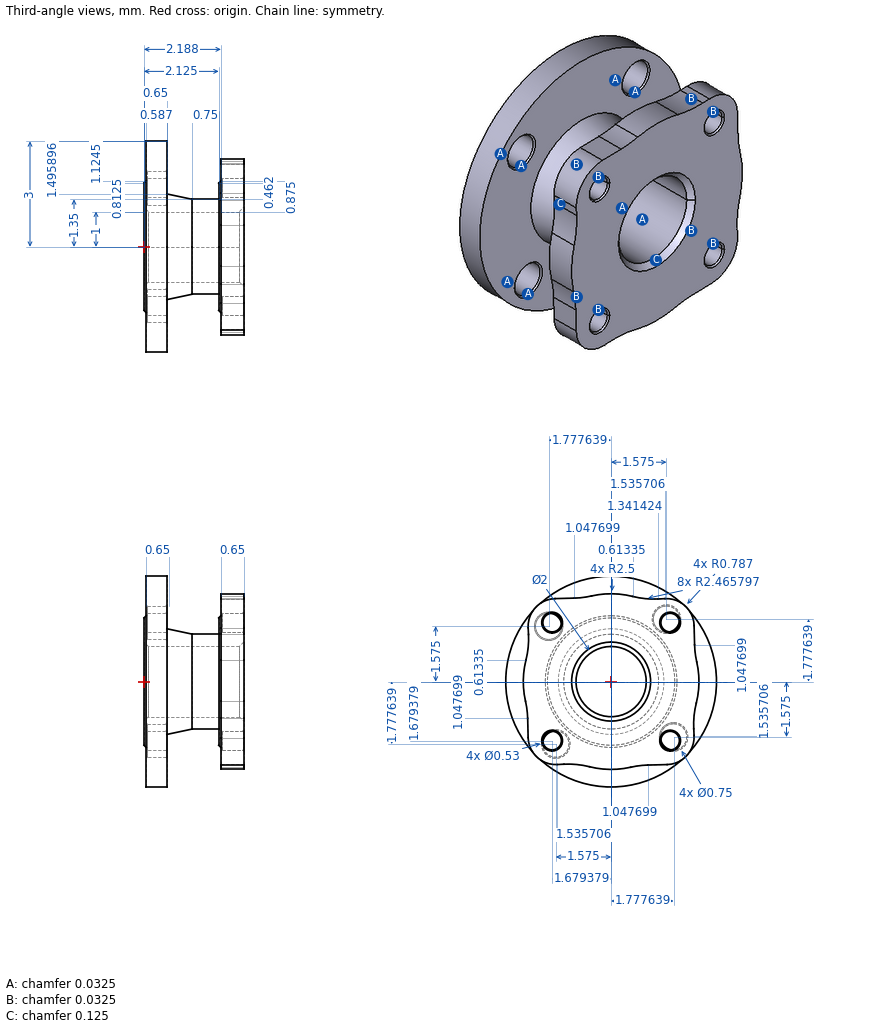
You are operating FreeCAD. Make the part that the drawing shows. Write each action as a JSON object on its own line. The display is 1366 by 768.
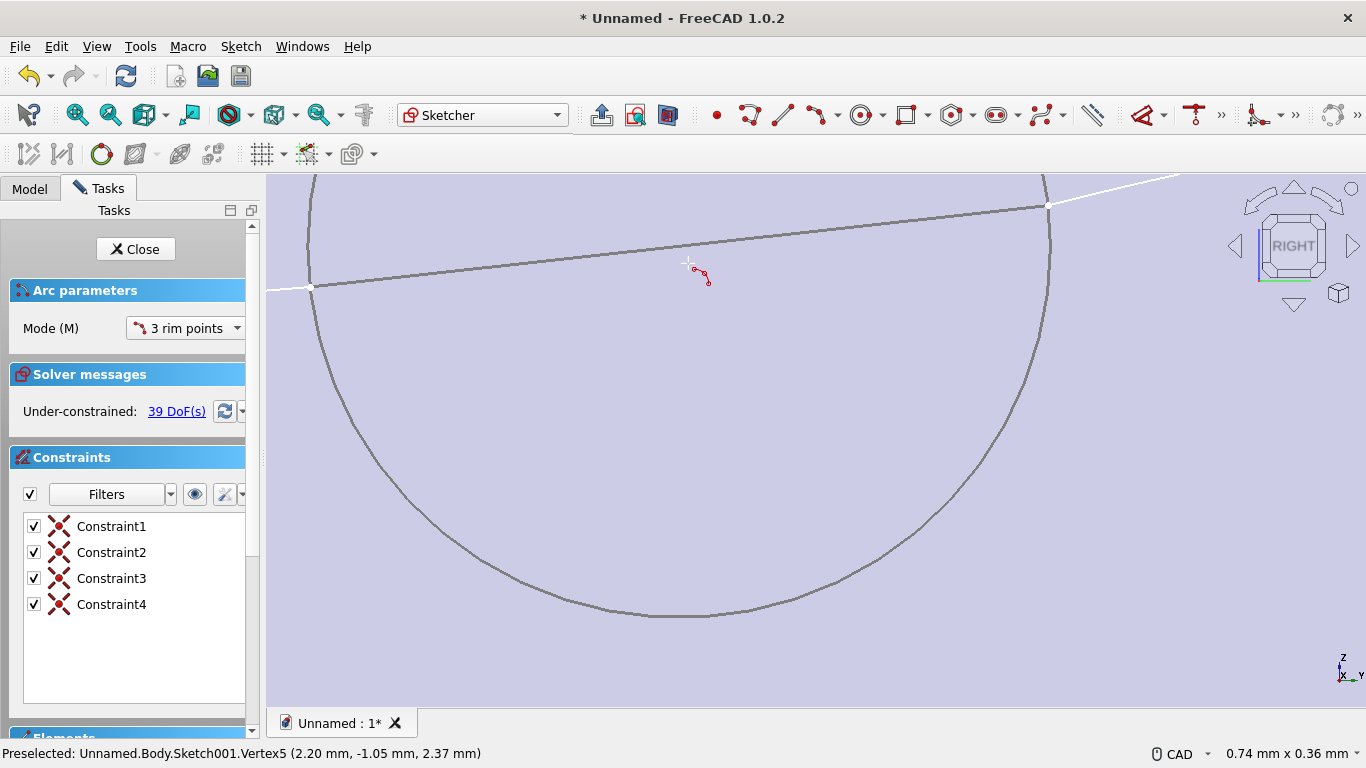
{"action": "left_click", "coordinate": [683, 250]}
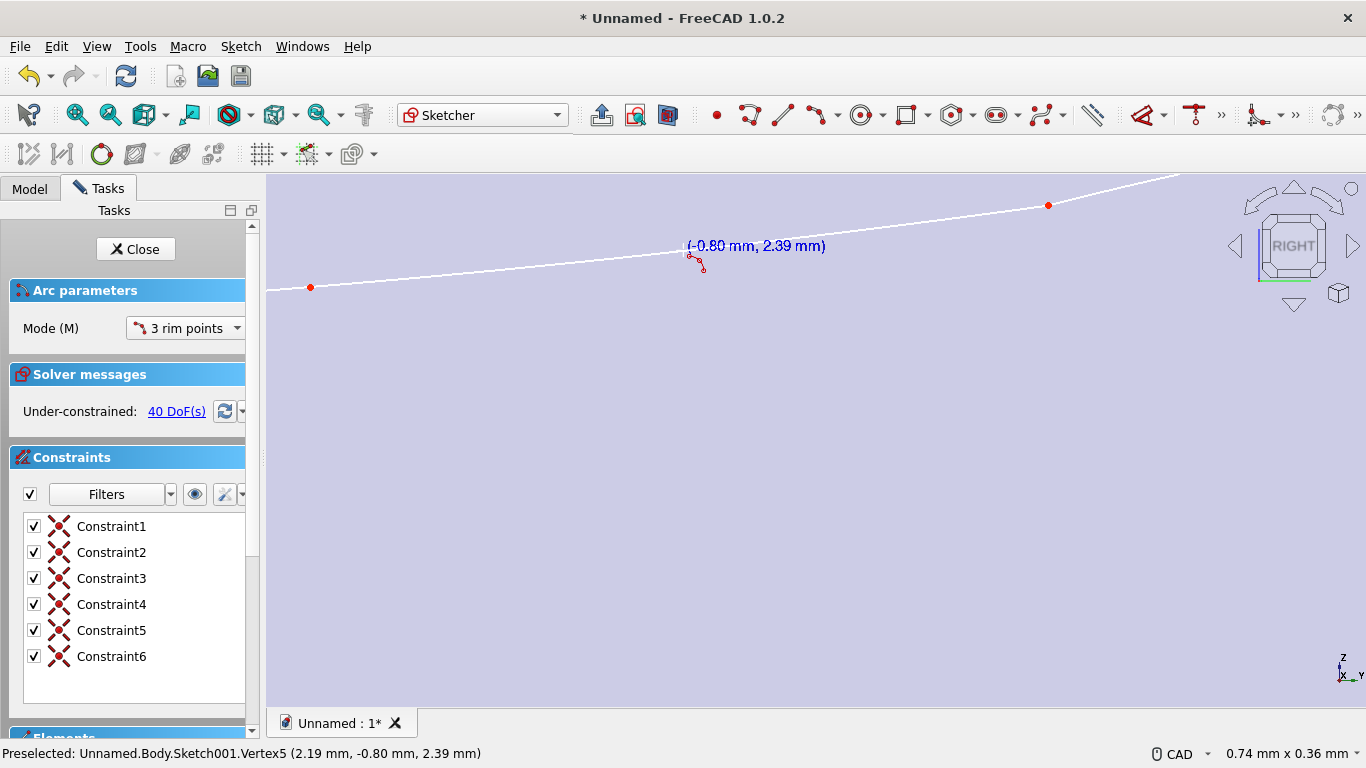
{"action": "scroll", "coordinate": [688, 263], "scroll_direction": "down", "scroll_amount": 15}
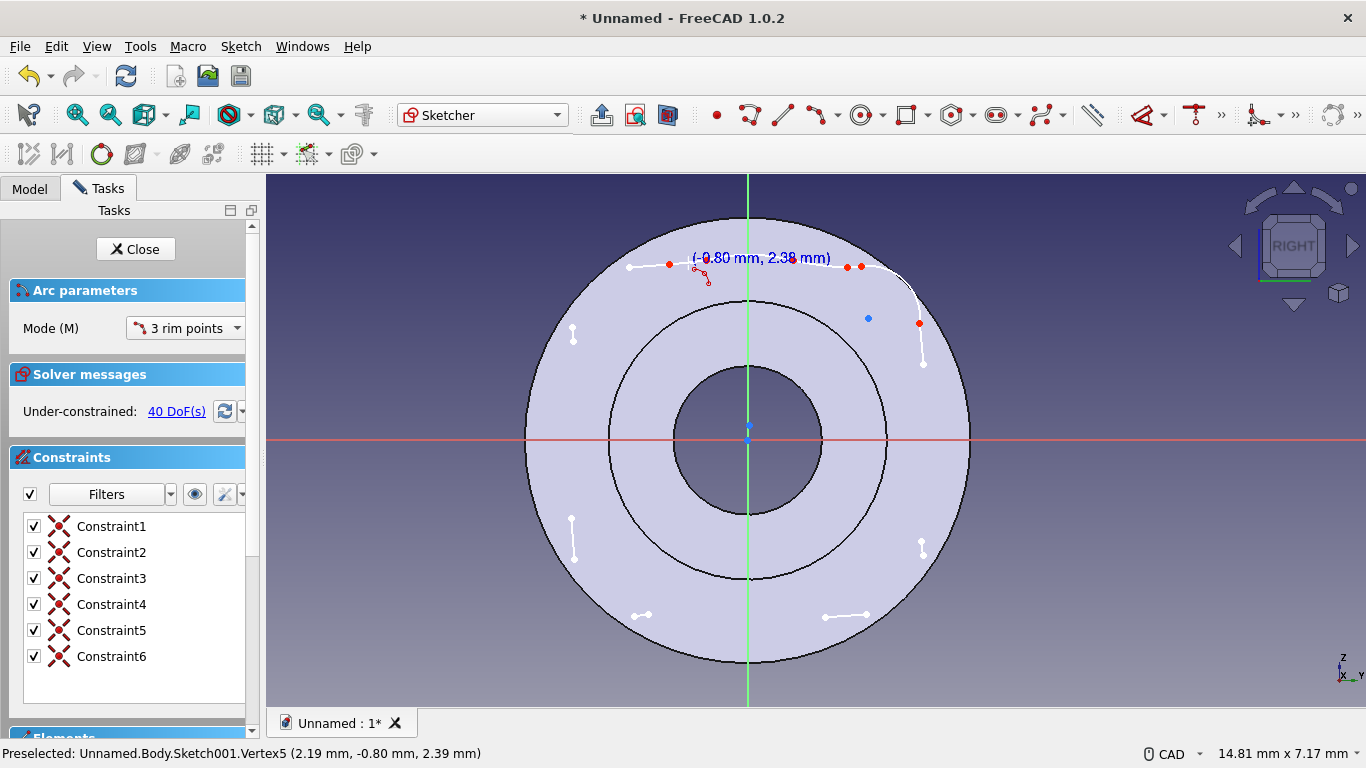
{"action": "left_click", "coordinate": [629, 268]}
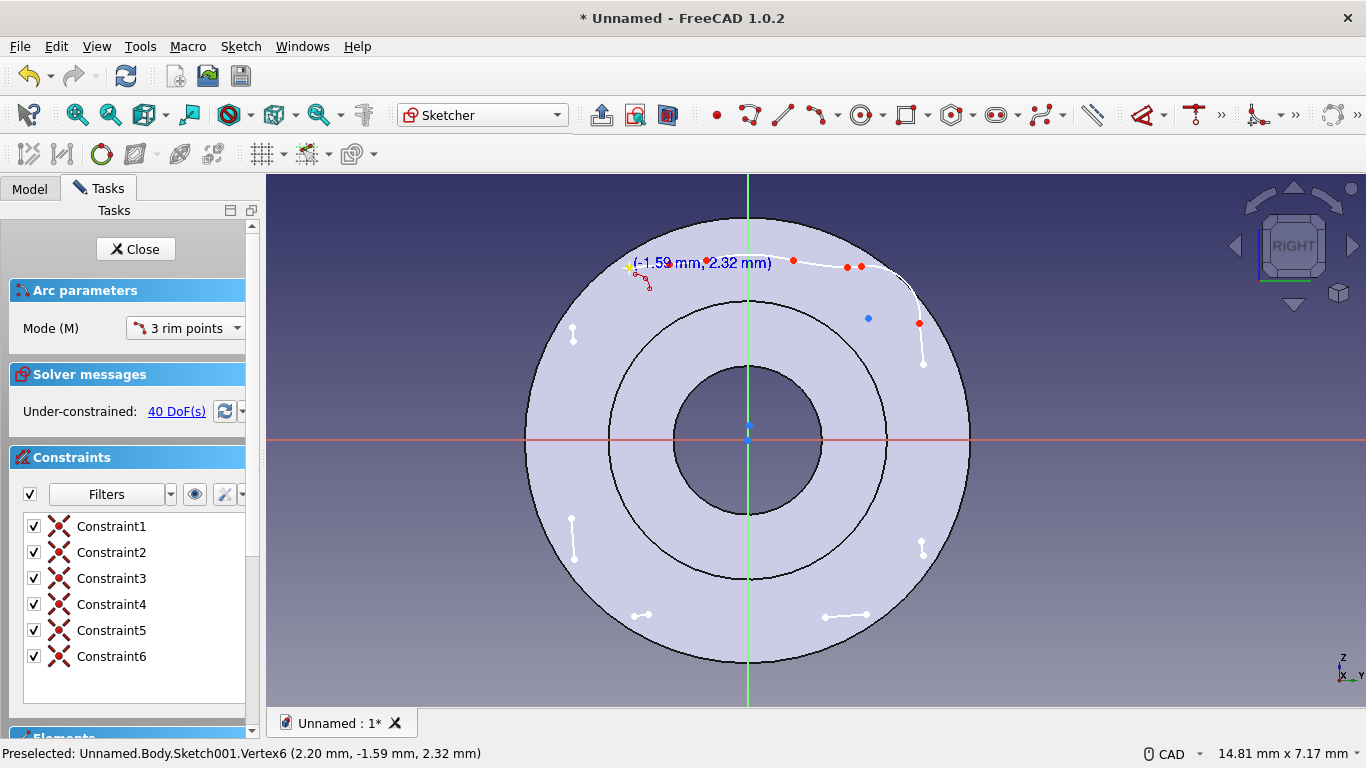
{"action": "scroll", "coordinate": [572, 326], "scroll_direction": "up", "scroll_amount": 4}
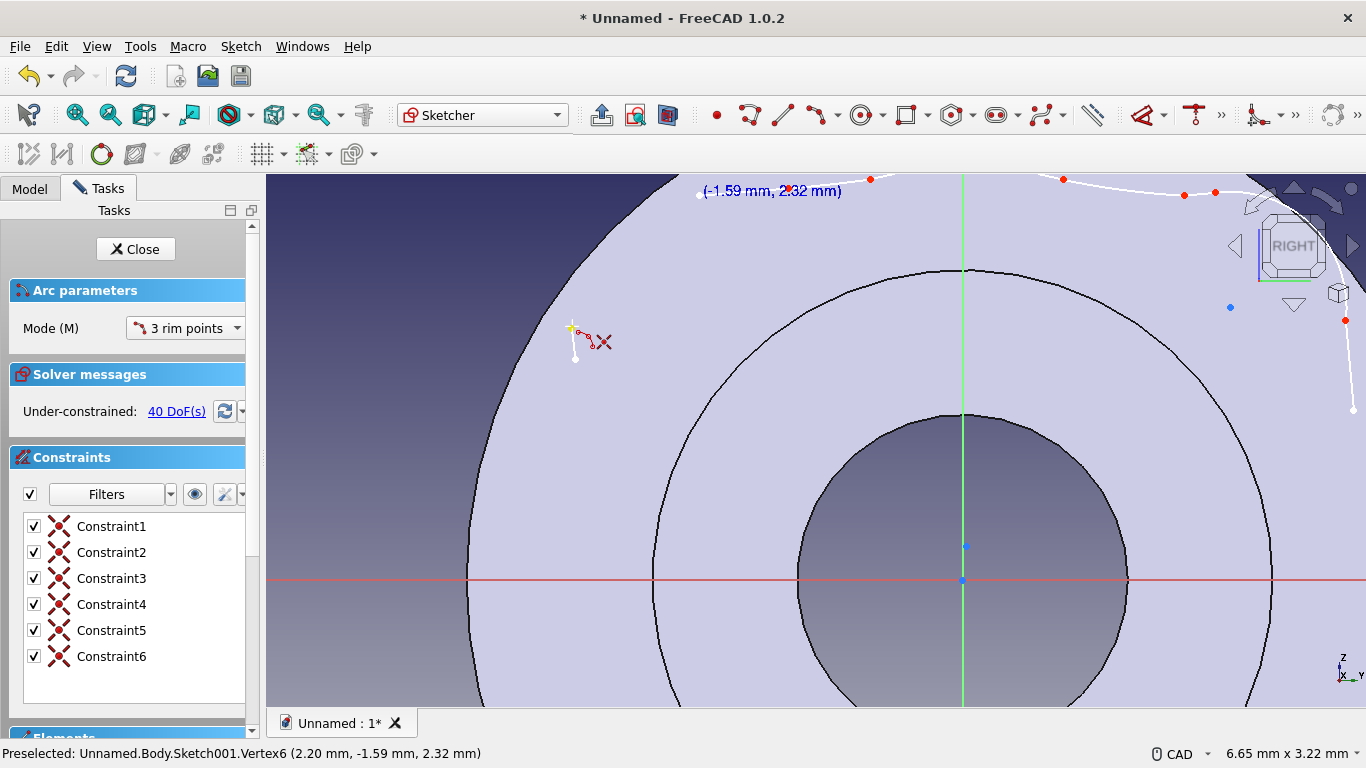
{"action": "left_click", "coordinate": [572, 329]}
{"action": "left_click", "coordinate": [607, 231]}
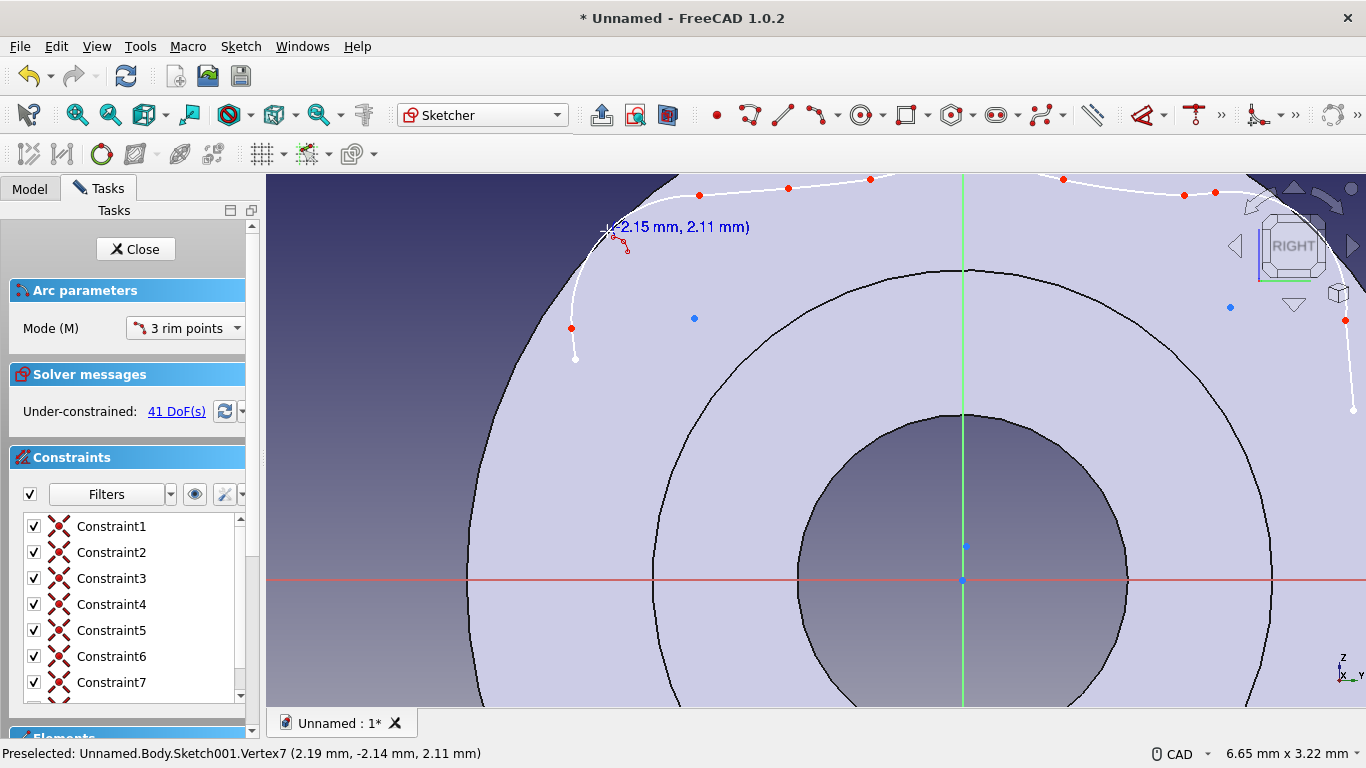
{"action": "left_click", "coordinate": [576, 360]}
{"action": "left_click", "coordinate": [562, 479]}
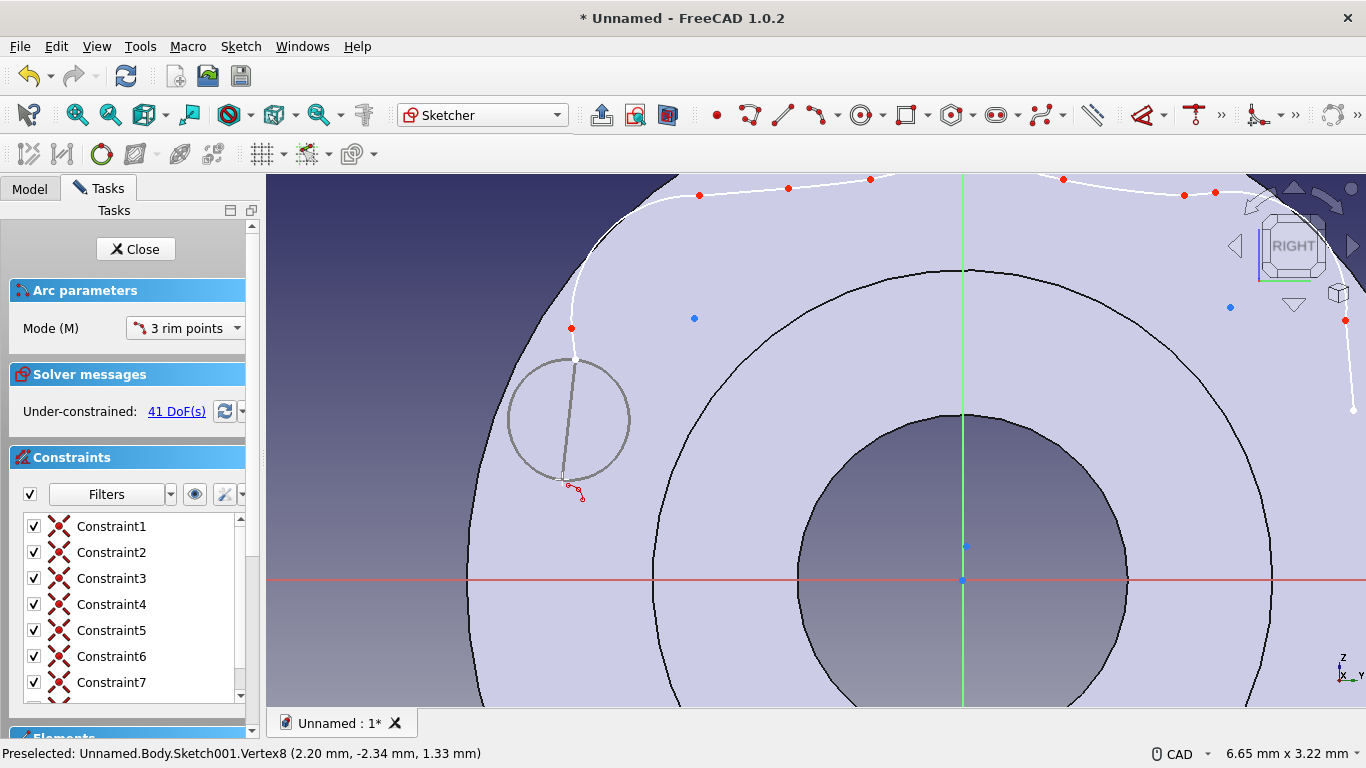
{"action": "scroll", "coordinate": [572, 419], "scroll_direction": "up", "scroll_amount": 7}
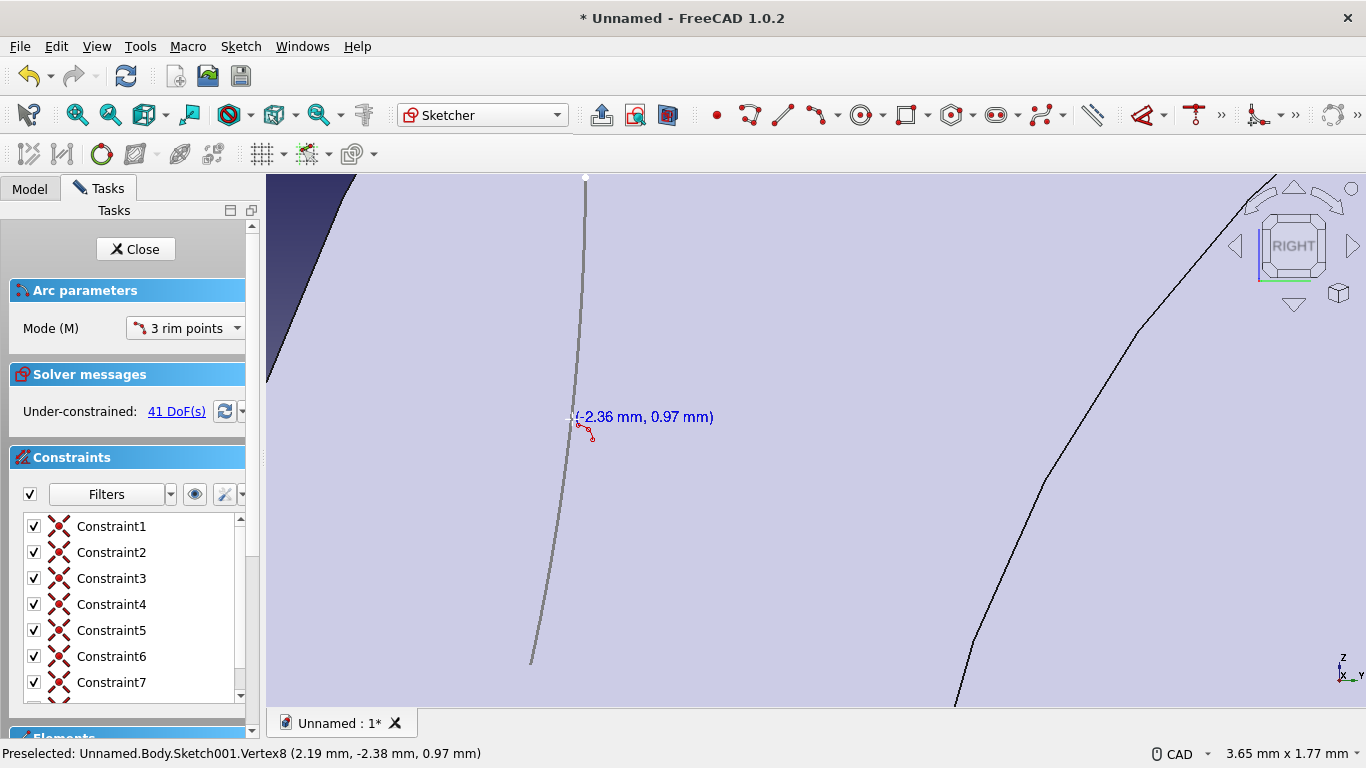
{"action": "left_click", "coordinate": [572, 418]}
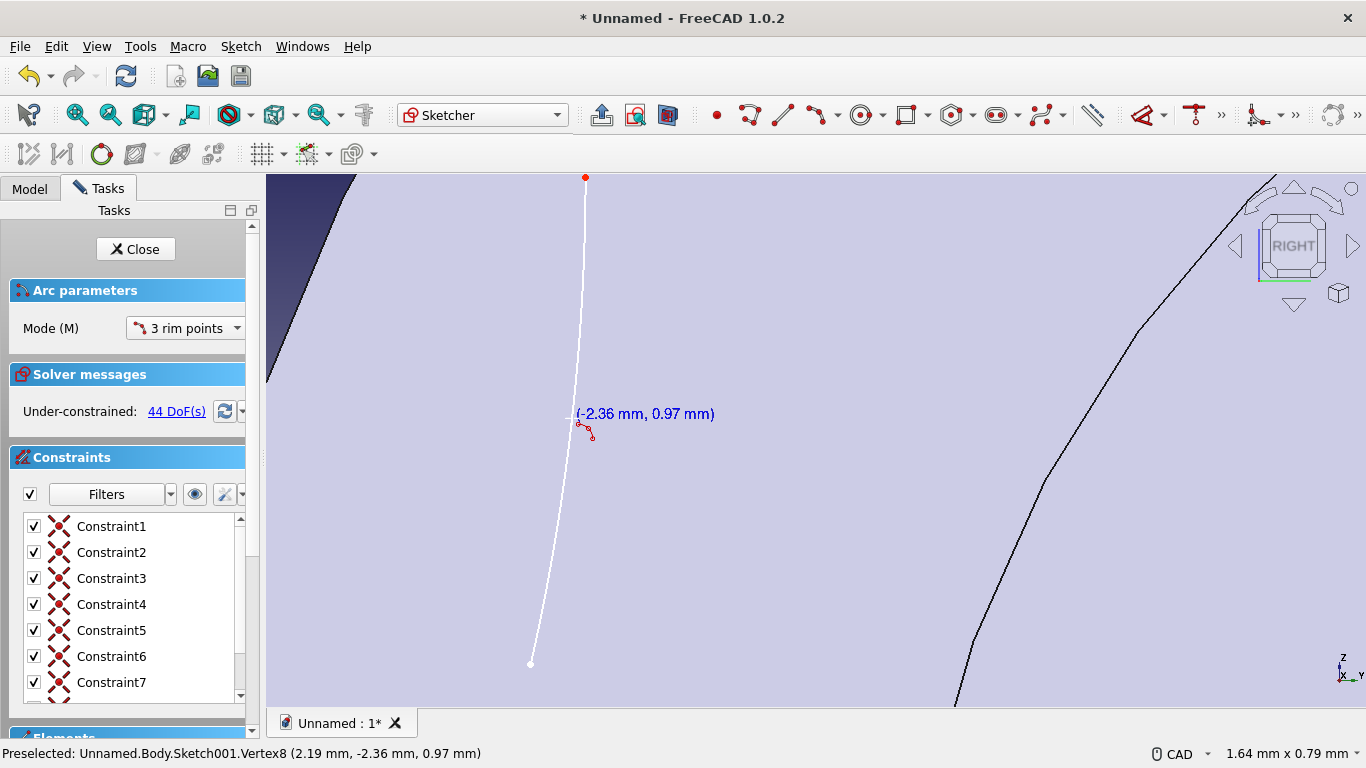
{"action": "scroll", "coordinate": [572, 362], "scroll_direction": "down", "scroll_amount": 11}